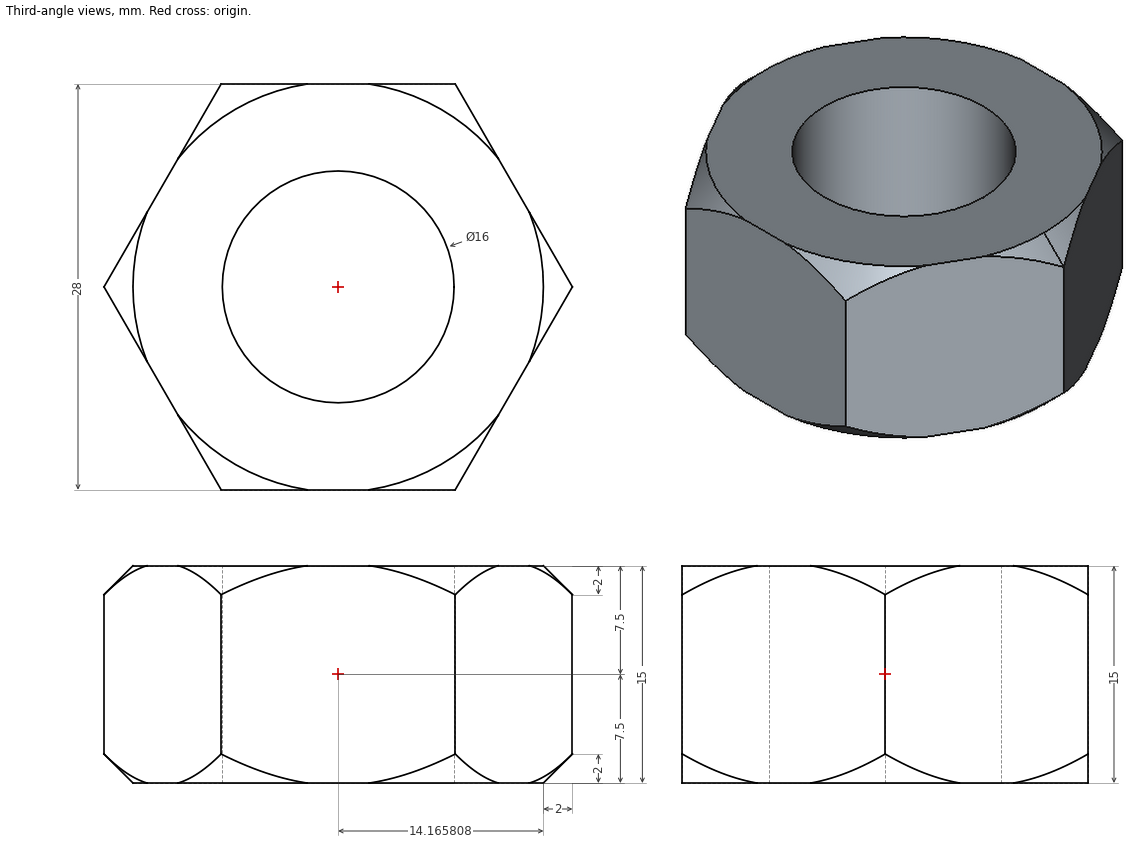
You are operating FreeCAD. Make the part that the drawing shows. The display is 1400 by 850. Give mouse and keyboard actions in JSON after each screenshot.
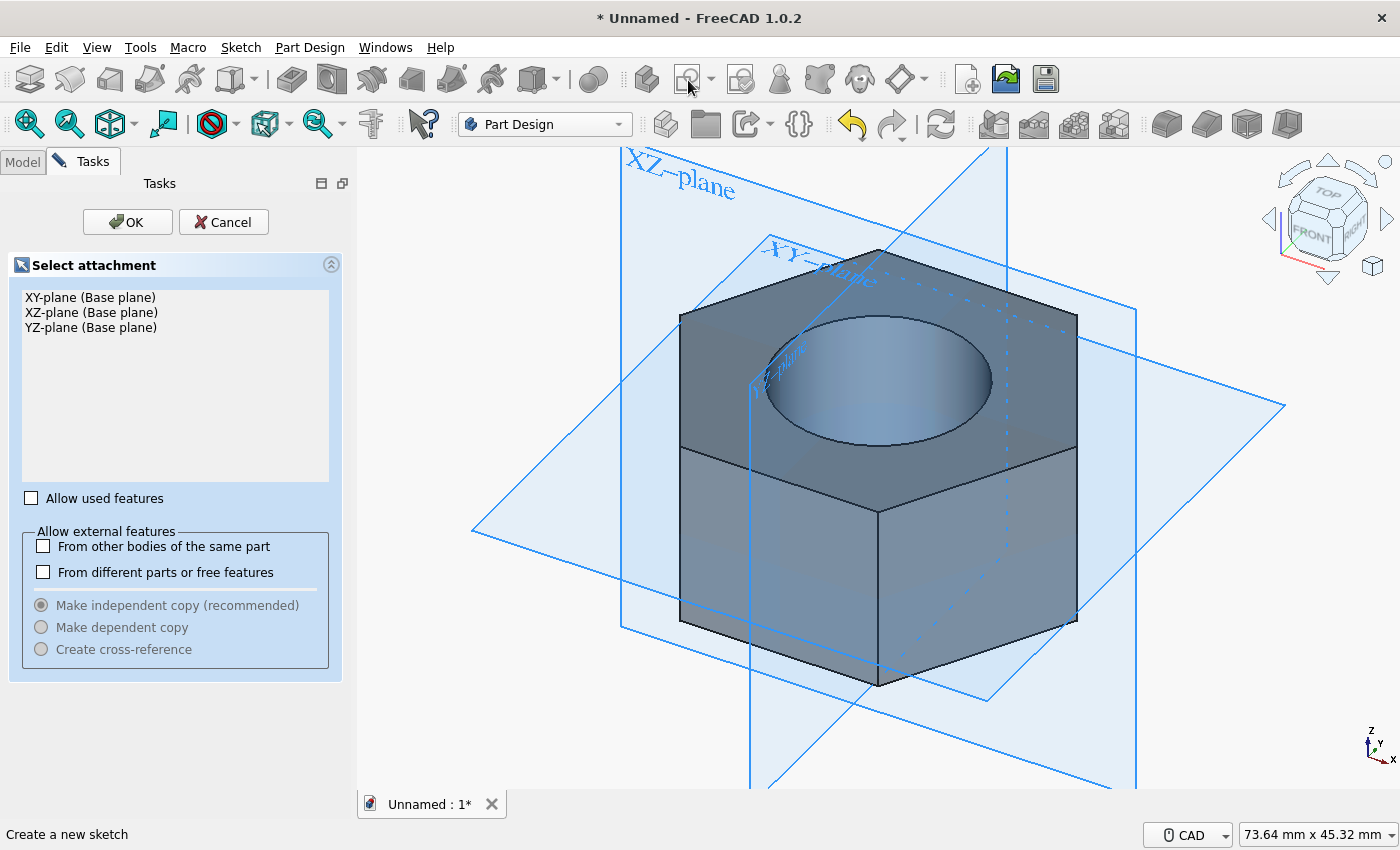
{"action": "left_click", "coordinate": [82, 312]}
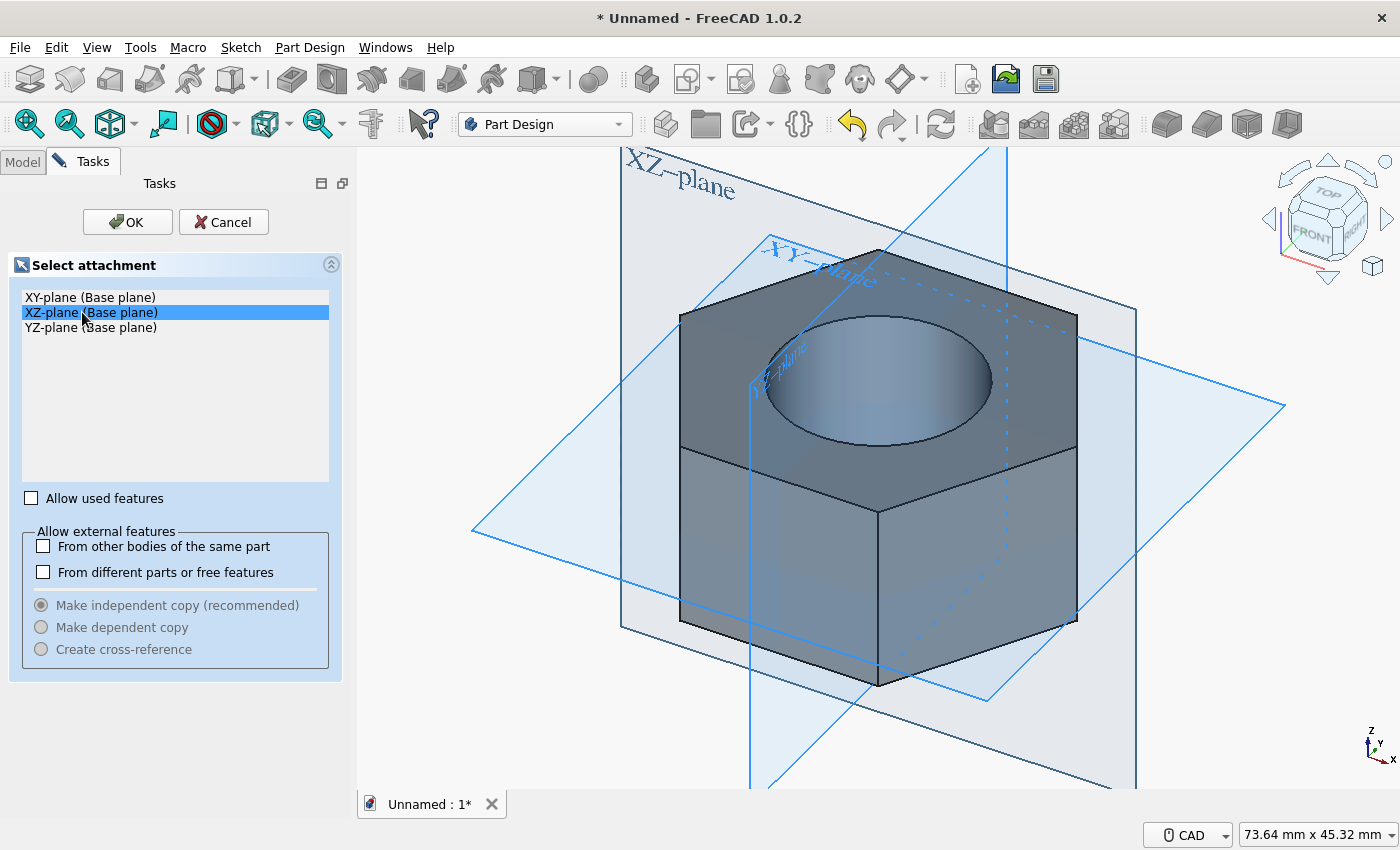
{"action": "left_click", "coordinate": [128, 222]}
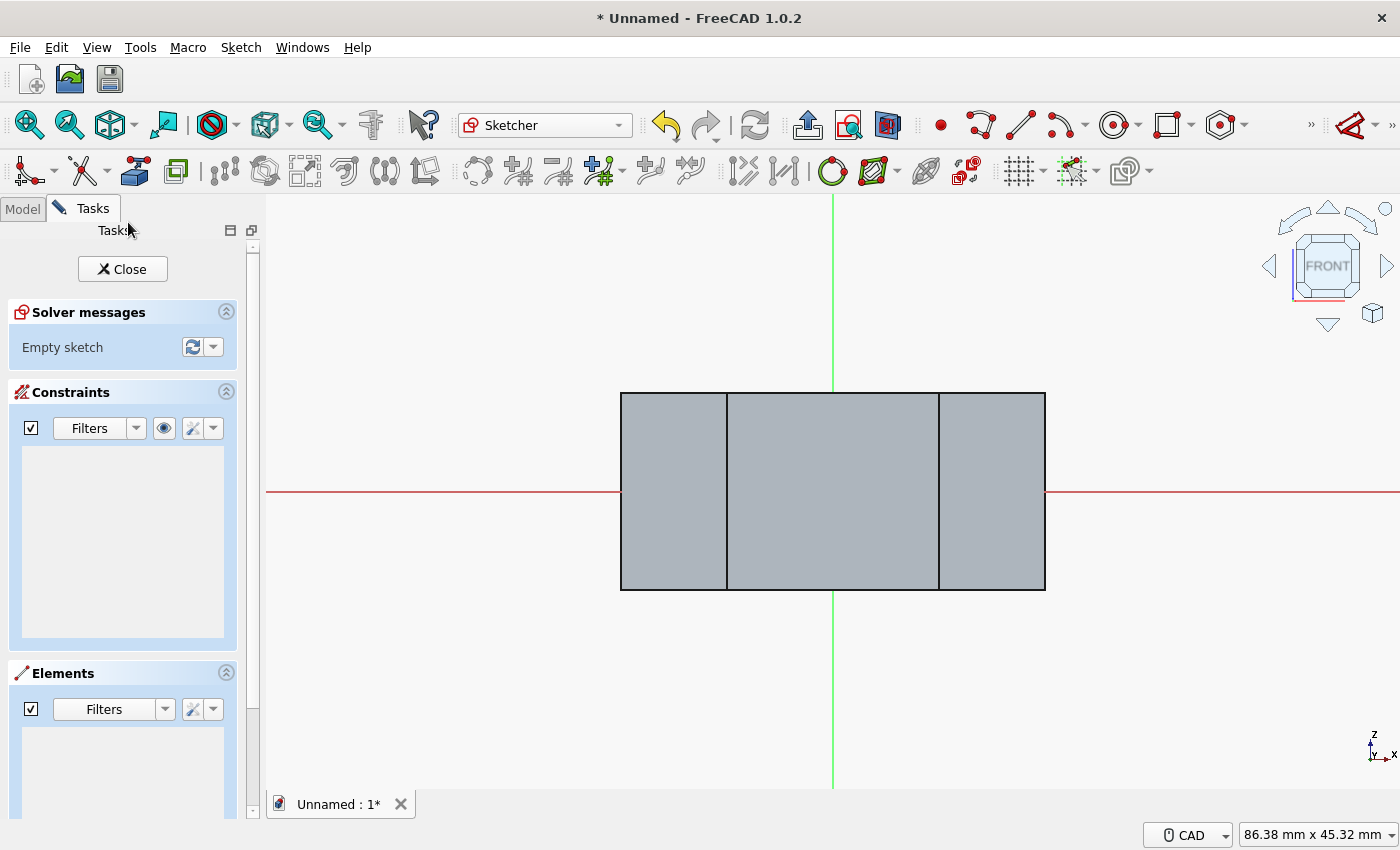
{"action": "left_click", "coordinate": [888, 126]}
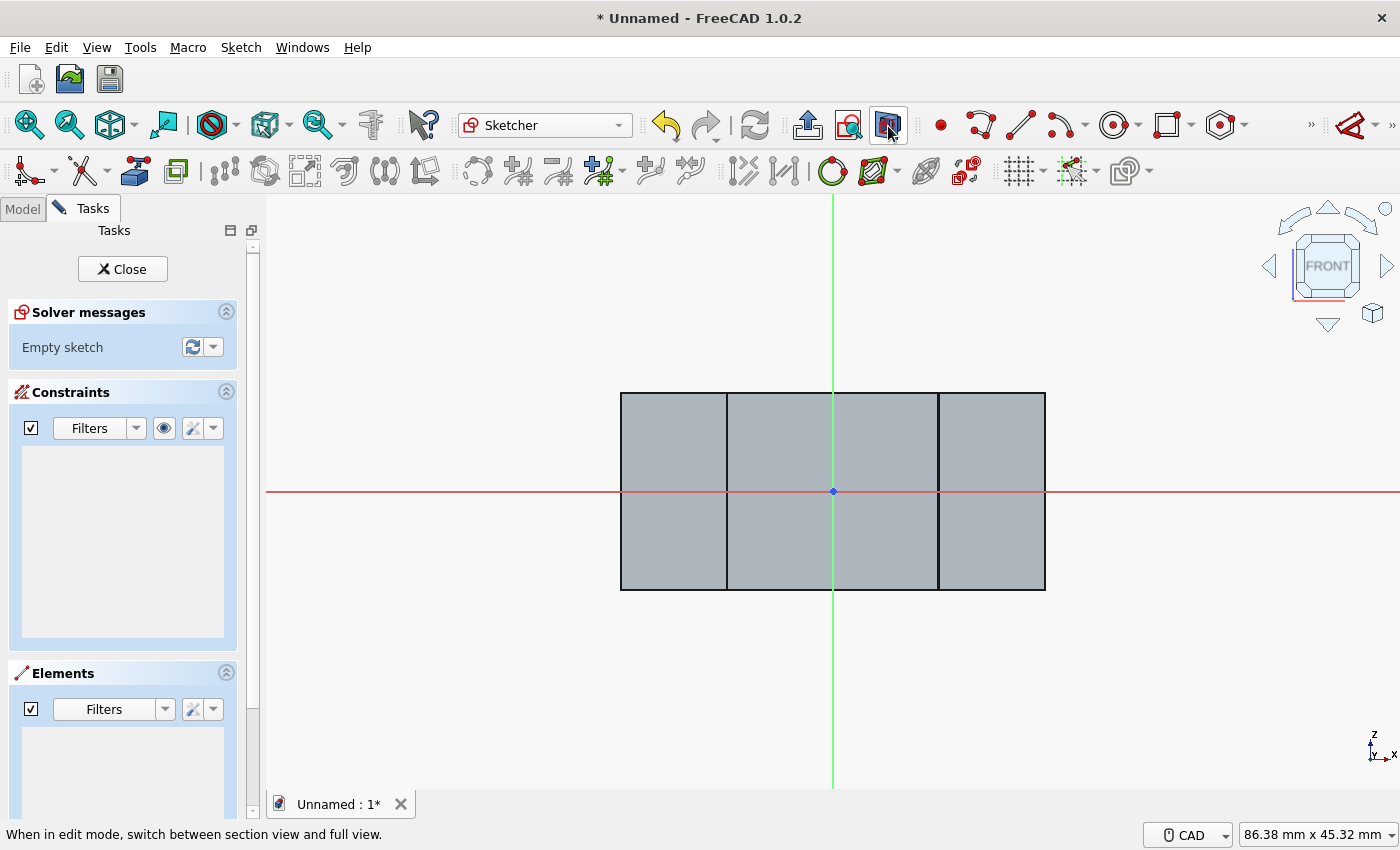
{"action": "scroll", "coordinate": [1151, 492], "scroll_direction": "up", "scroll_amount": 3}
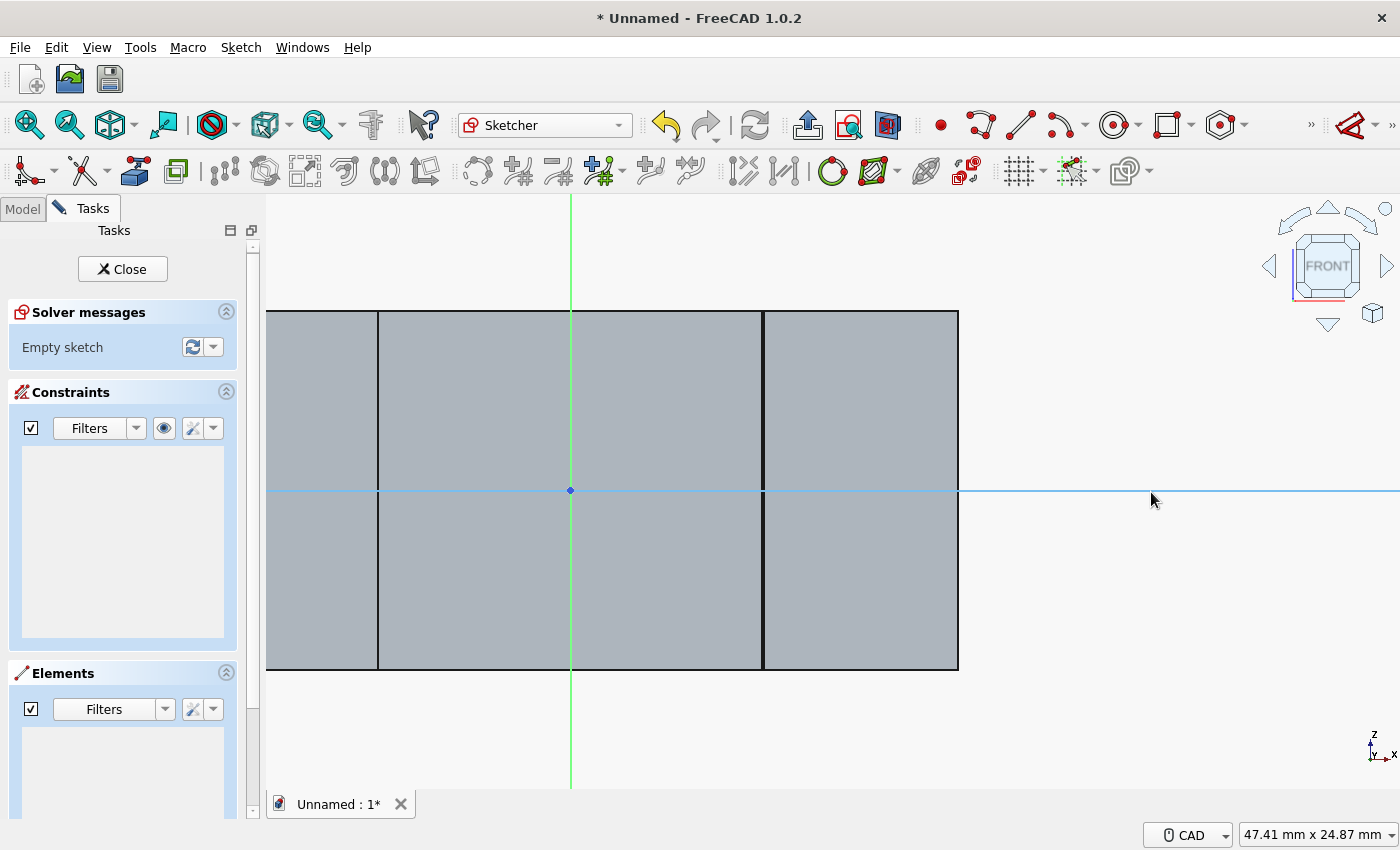
{"action": "left_click", "coordinate": [982, 126]}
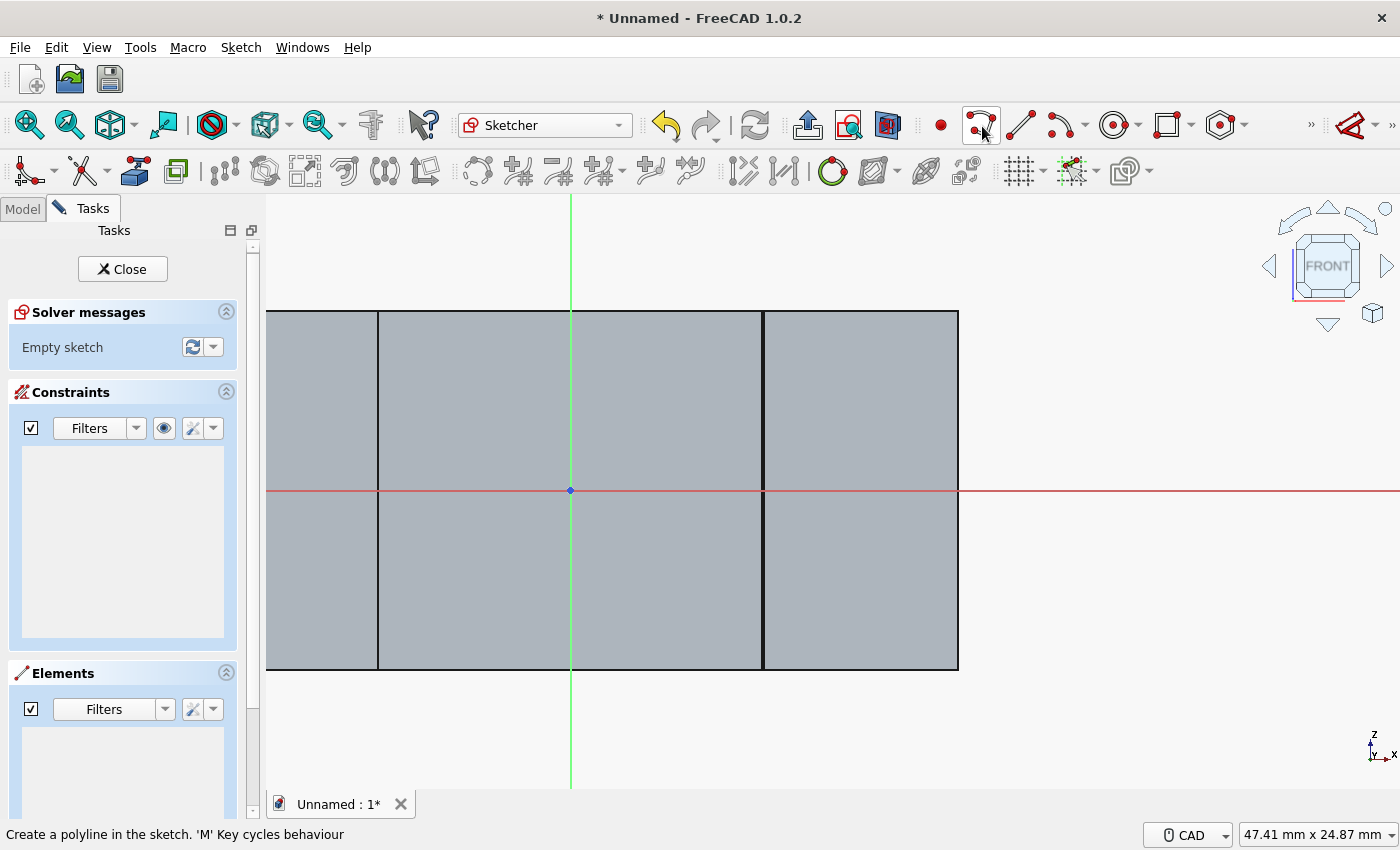
{"action": "left_click", "coordinate": [910, 670]}
{"action": "left_click", "coordinate": [958, 622]}
{"action": "left_click", "coordinate": [958, 670]}
{"action": "left_click", "coordinate": [910, 671]}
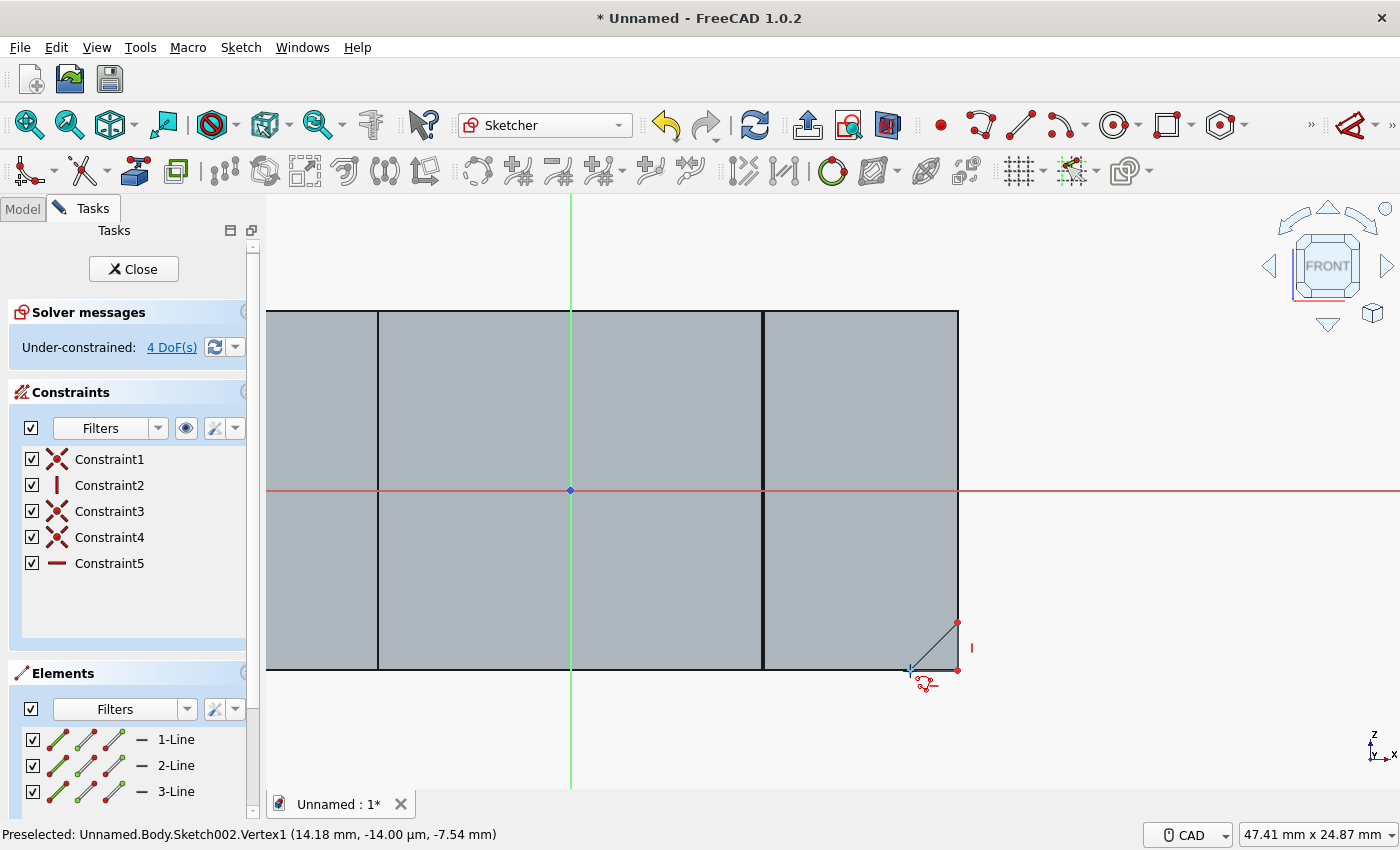
{"action": "left_click", "coordinate": [910, 311]}
{"action": "left_click", "coordinate": [958, 311]}
{"action": "left_click", "coordinate": [958, 359]}
{"action": "left_click", "coordinate": [910, 312]}
{"action": "key", "text": "Escape"}
{"action": "key", "text": "Escape"}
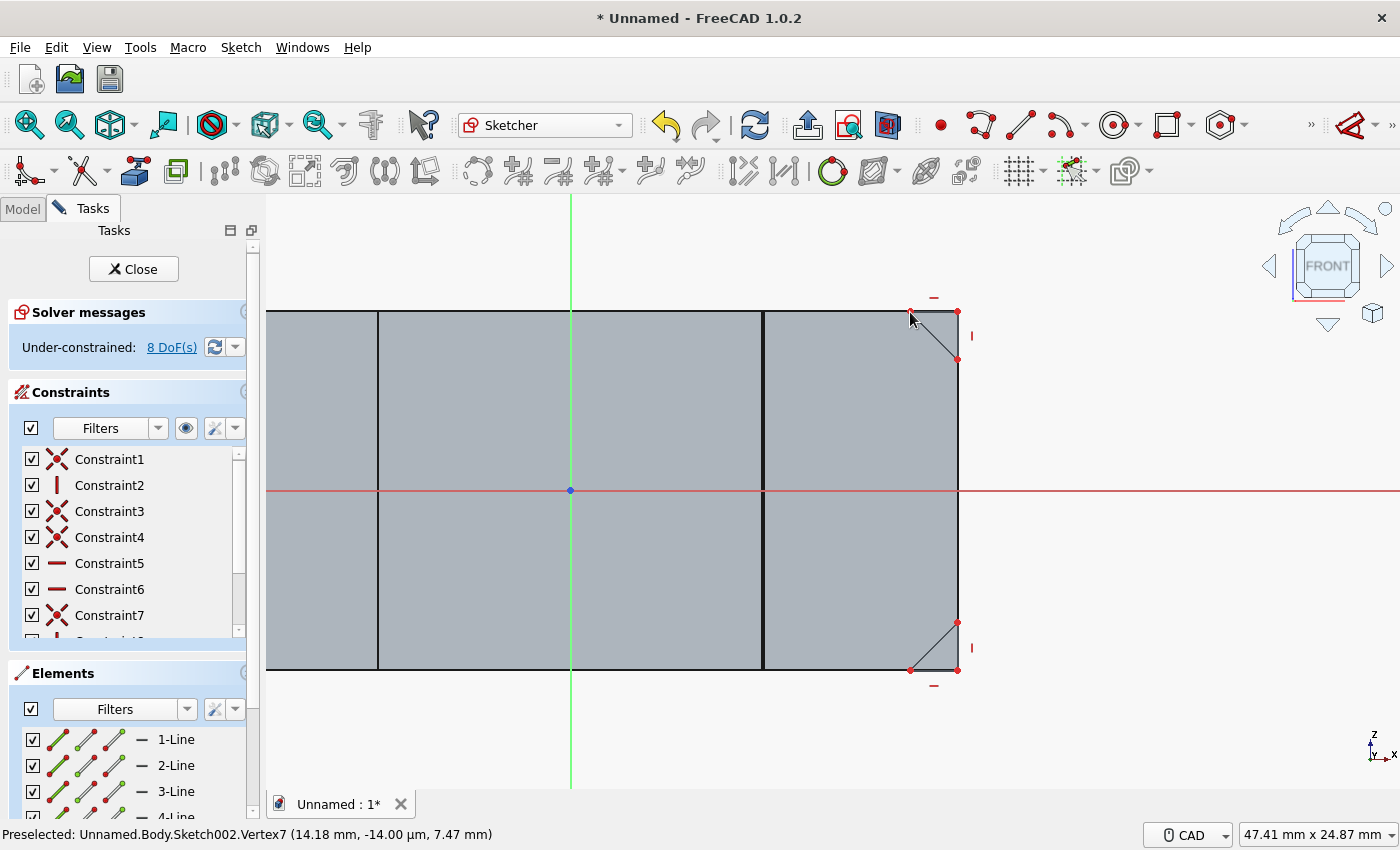
{"action": "left_click", "coordinate": [1350, 126]}